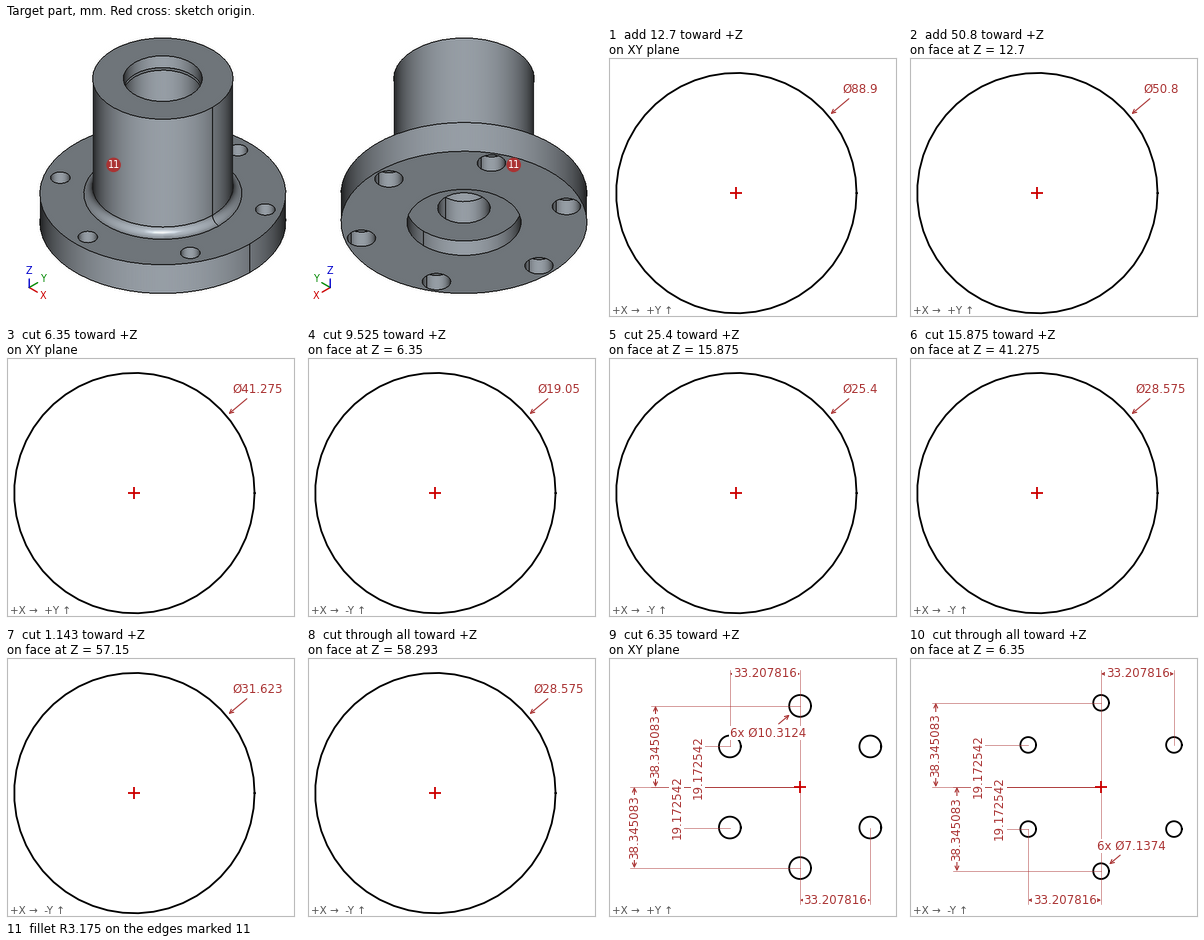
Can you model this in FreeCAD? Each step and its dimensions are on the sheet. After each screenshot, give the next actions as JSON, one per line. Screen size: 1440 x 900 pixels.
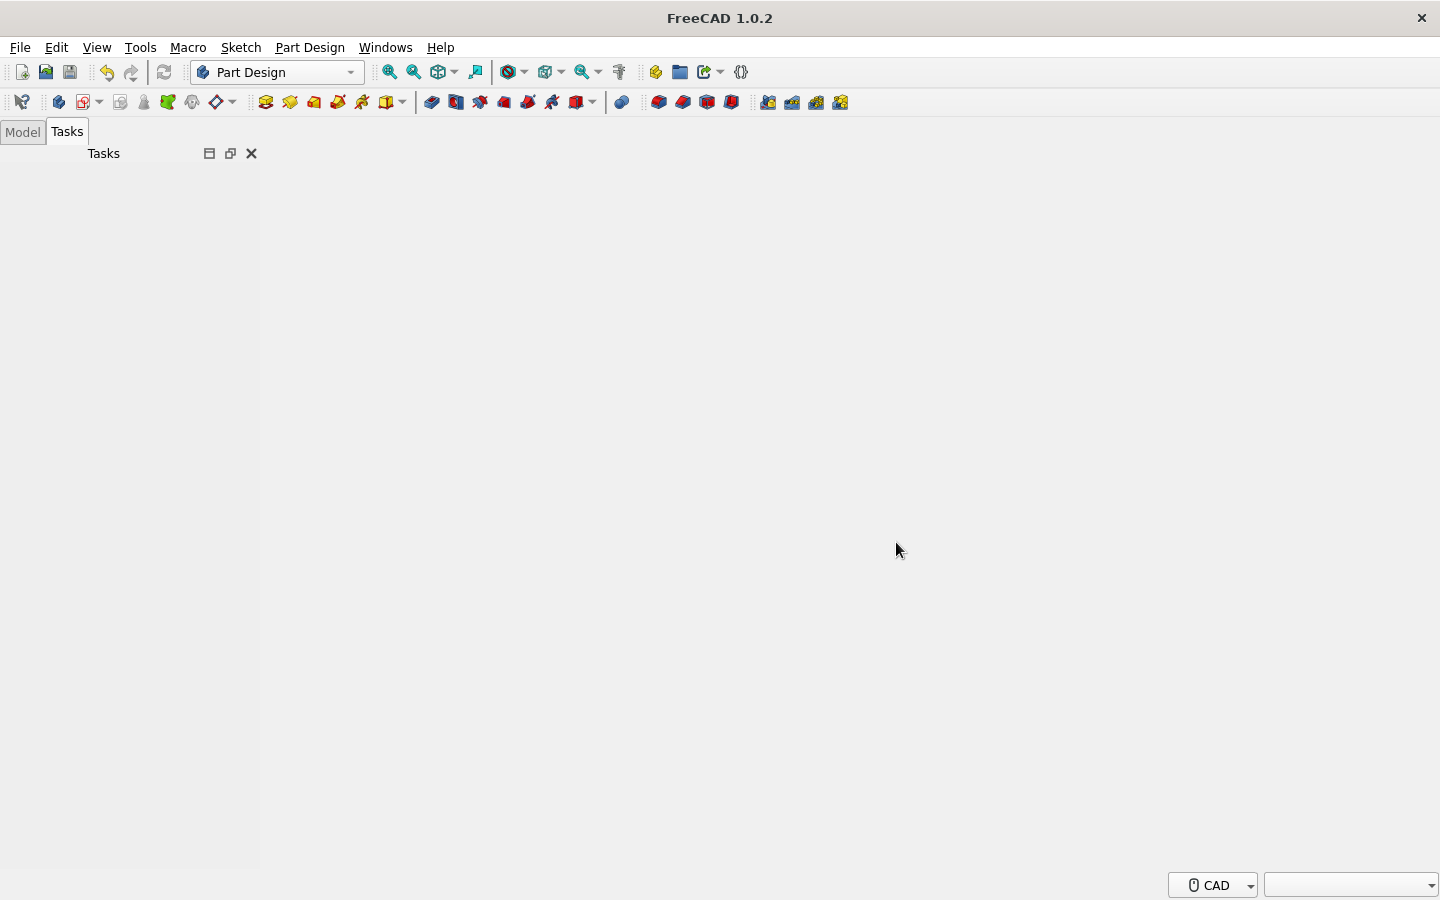
{"action": "left_click", "coordinate": [22, 72]}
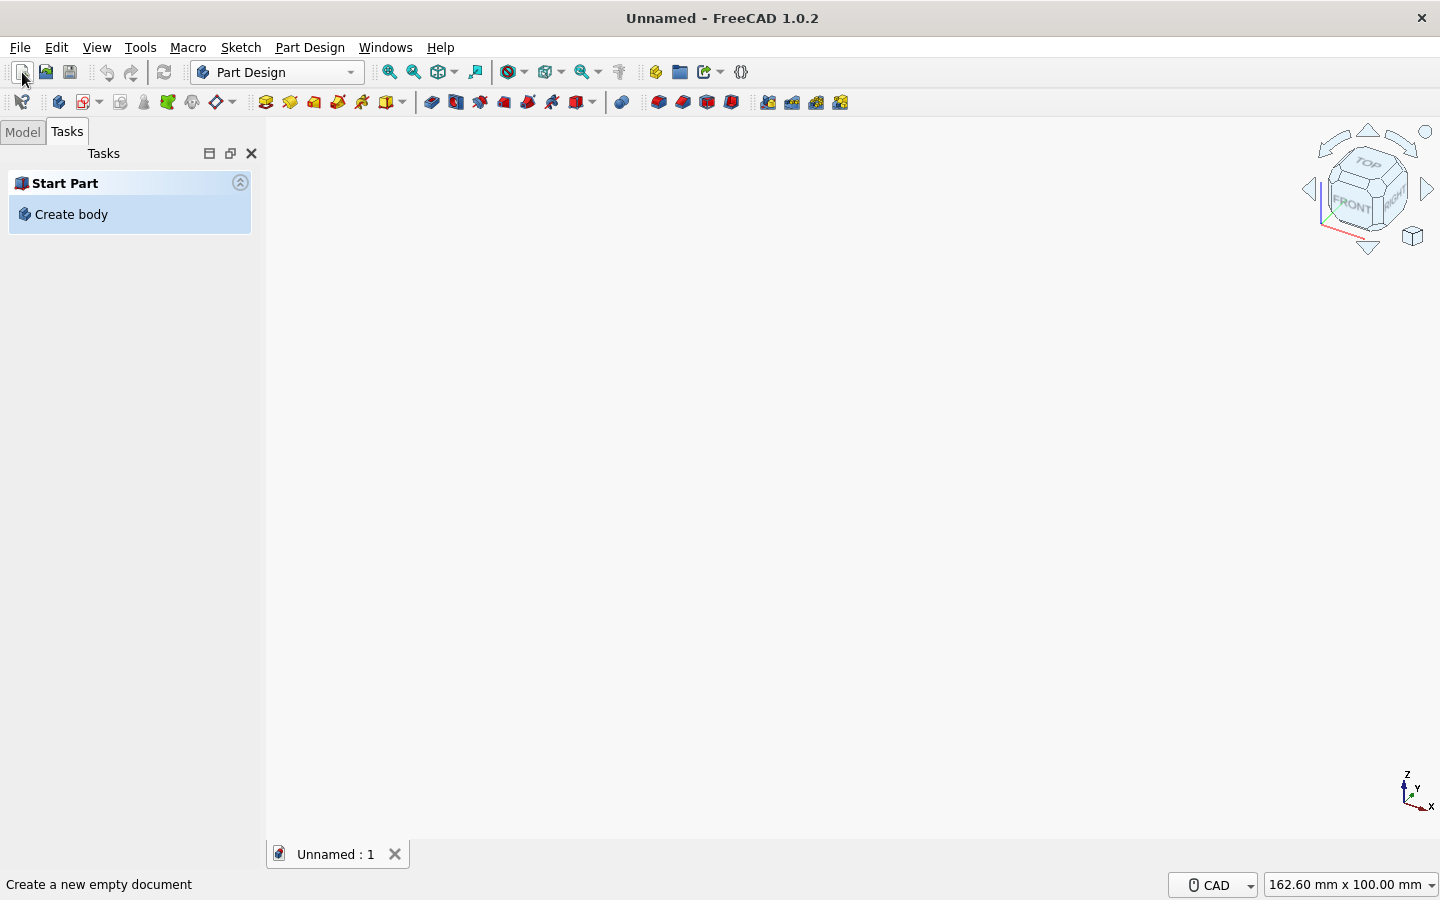
{"action": "left_click", "coordinate": [84, 102]}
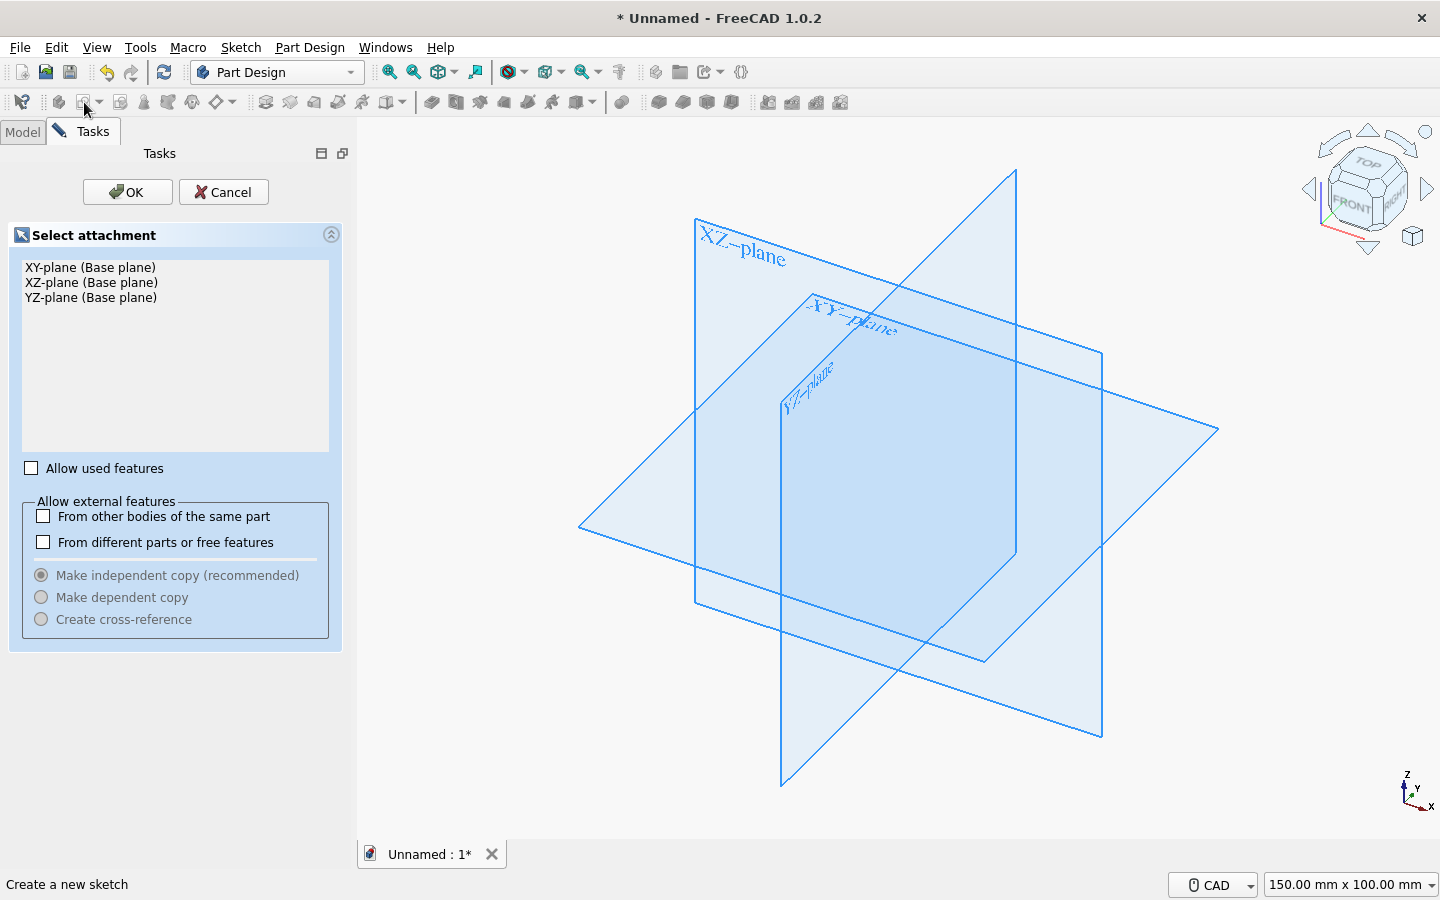
{"action": "left_click", "coordinate": [82, 268]}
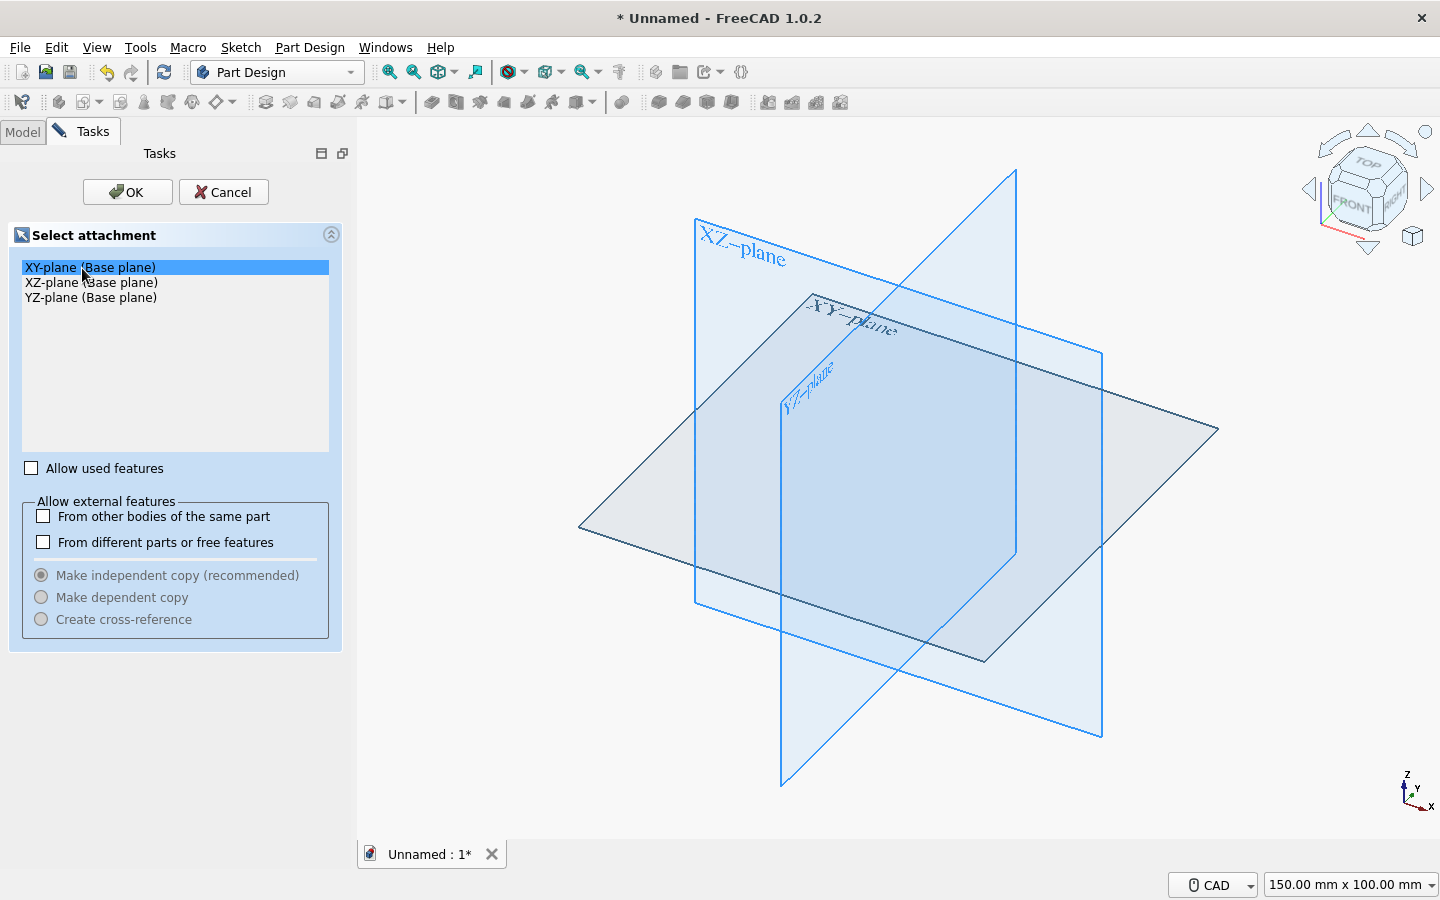
{"action": "left_click", "coordinate": [128, 192]}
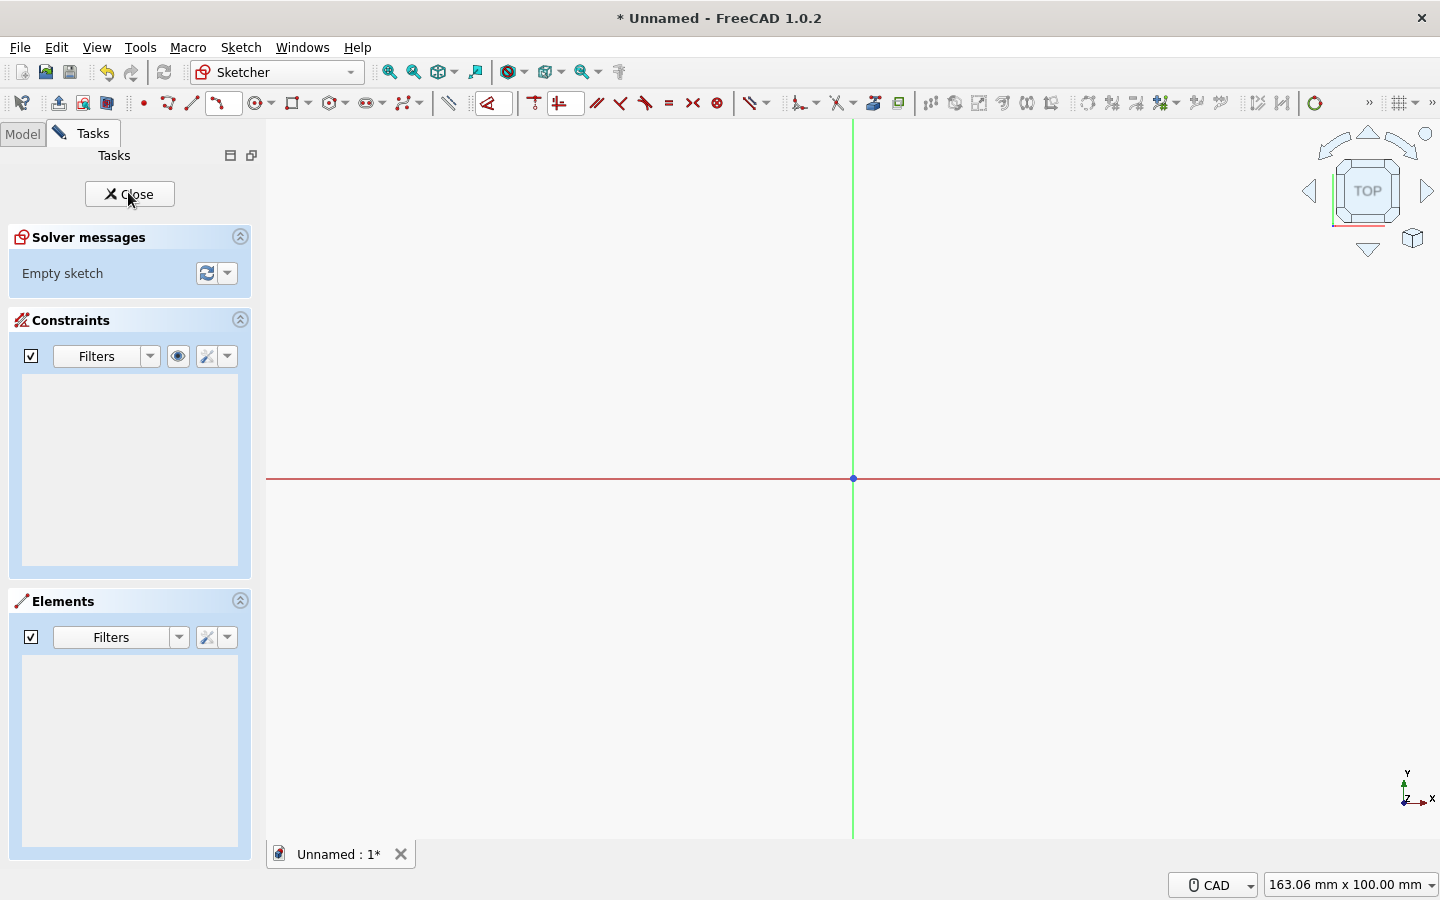
{"action": "scroll", "coordinate": [645, 479], "scroll_direction": "down", "scroll_amount": 2}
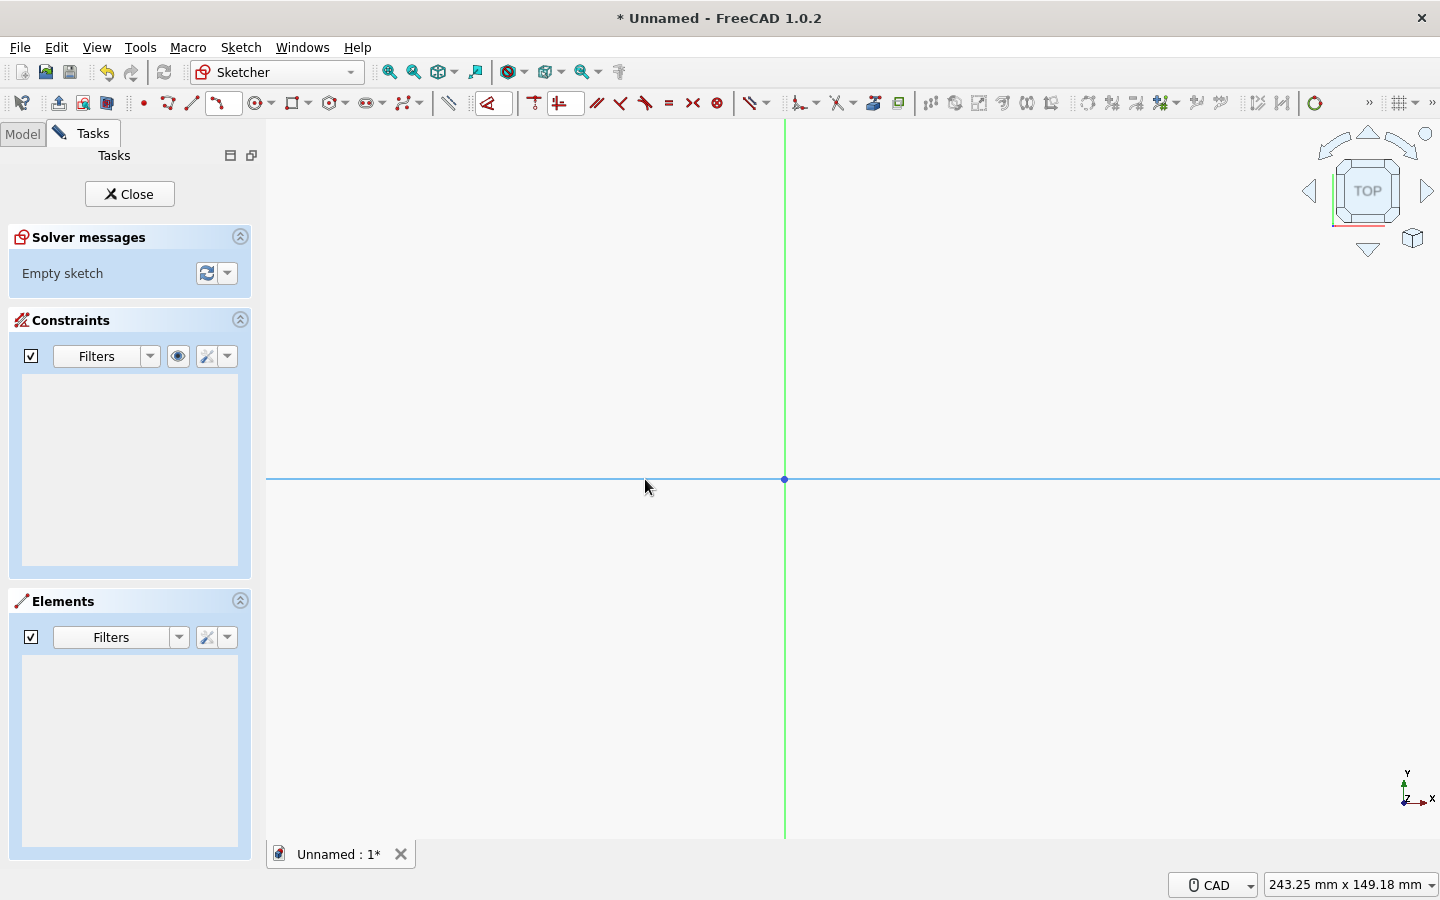
{"action": "left_click", "coordinate": [256, 104]}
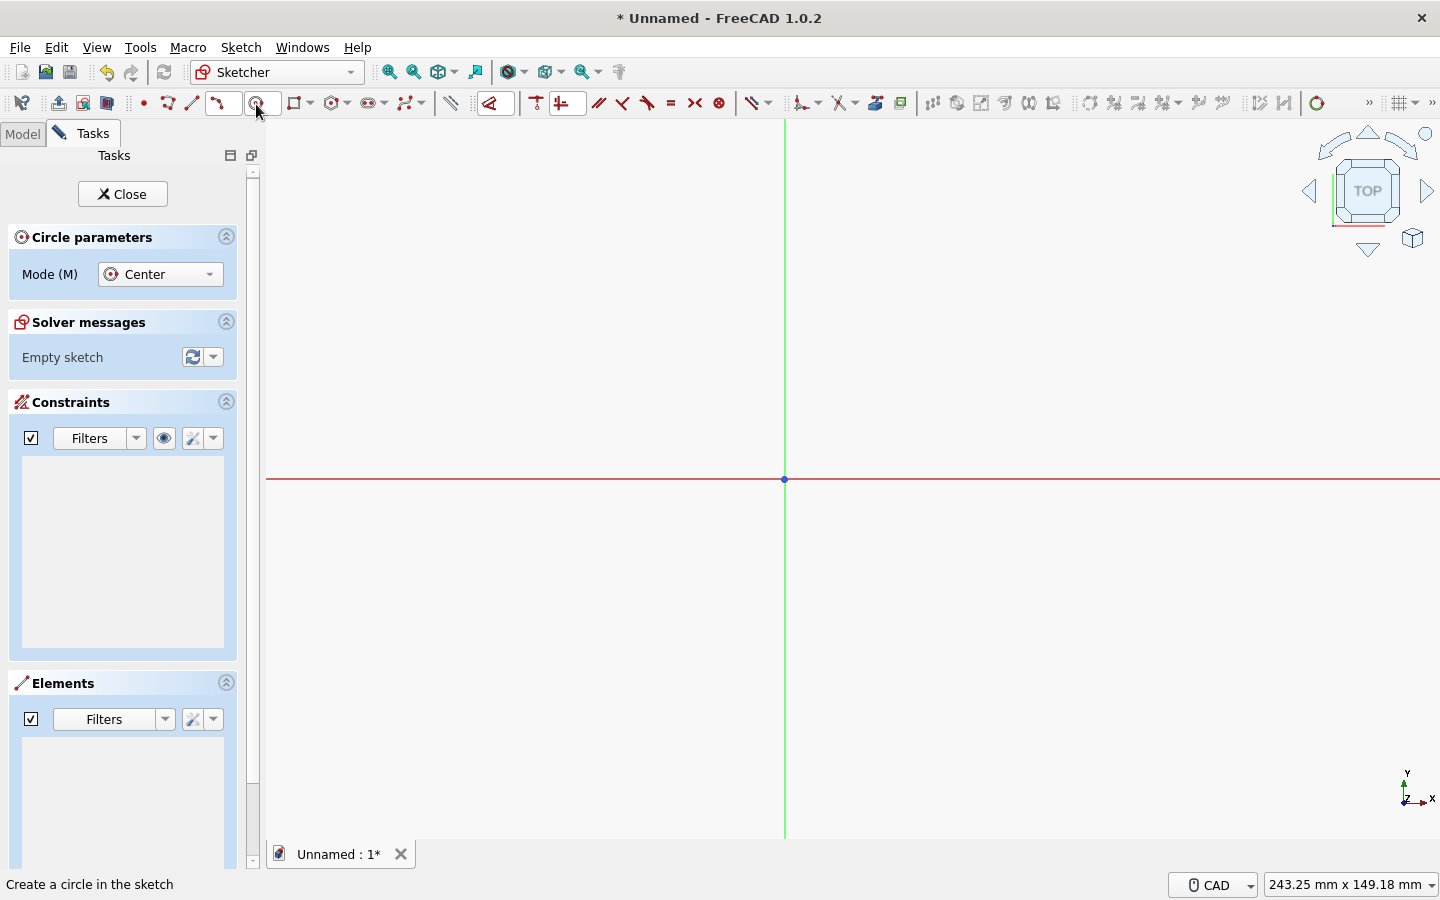
{"action": "left_click", "coordinate": [785, 479]}
{"action": "mouse_move", "coordinate": [936, 327]}